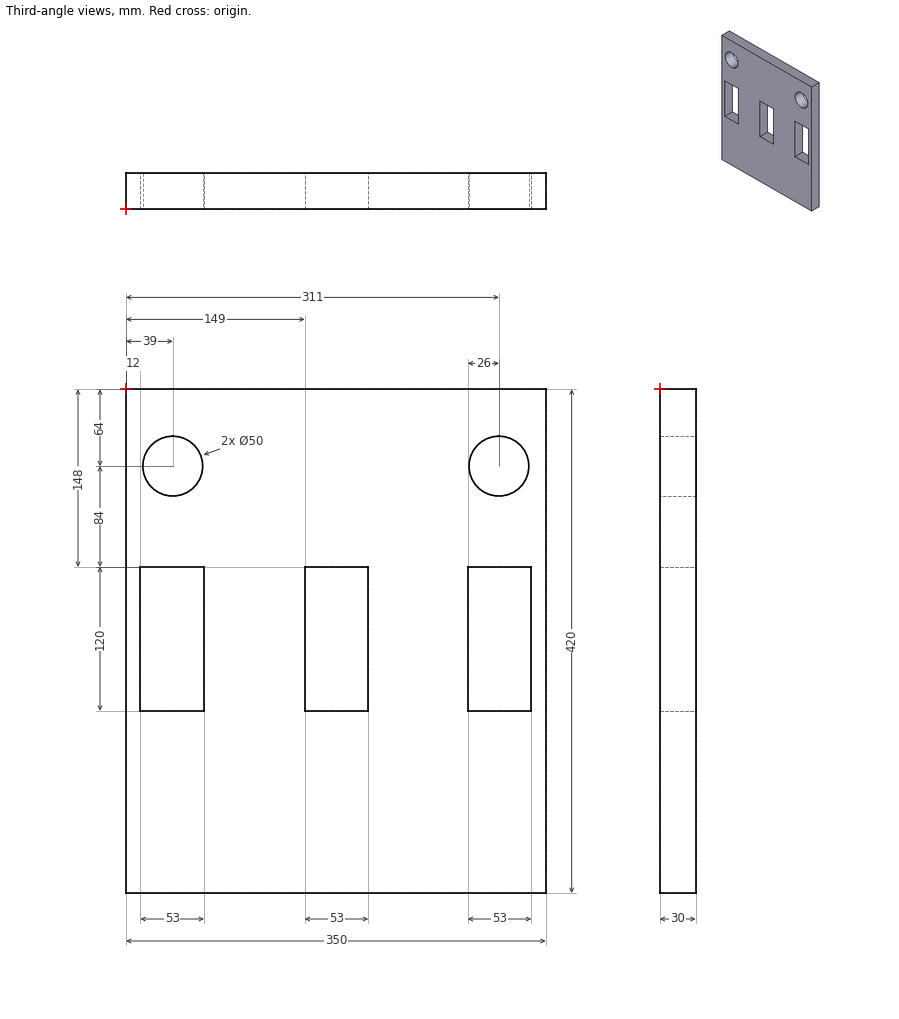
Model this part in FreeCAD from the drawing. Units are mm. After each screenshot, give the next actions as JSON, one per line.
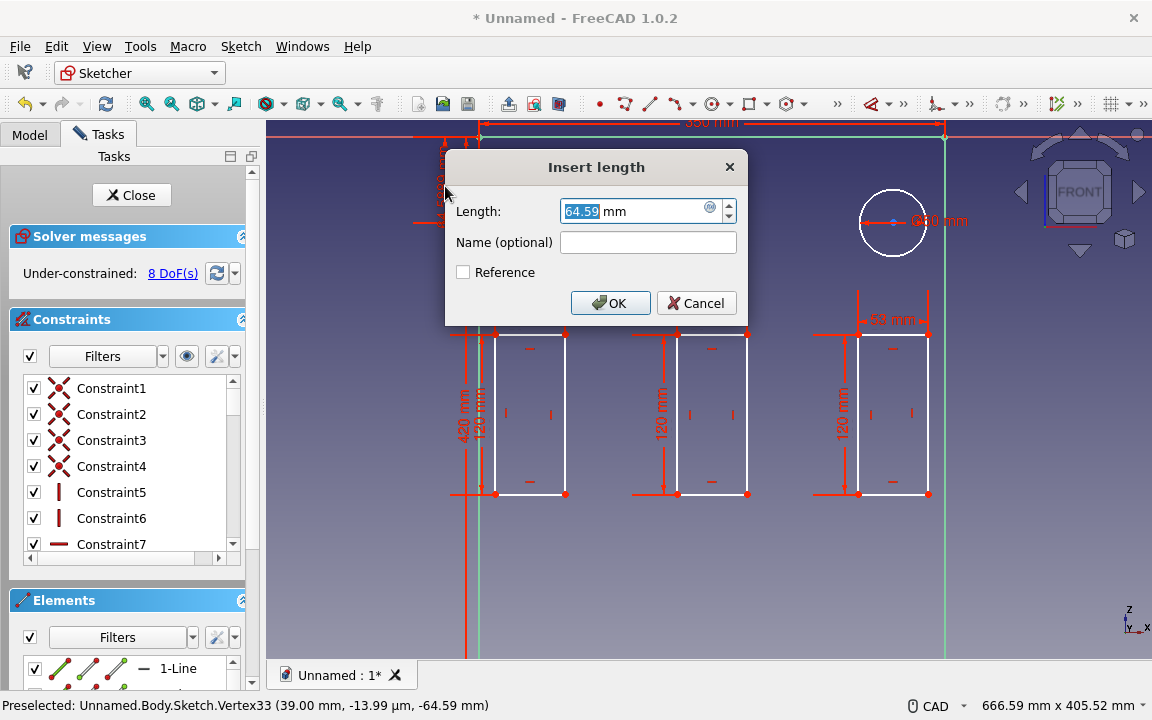
{"action": "type", "text": "64"}
{"action": "key", "text": "Return"}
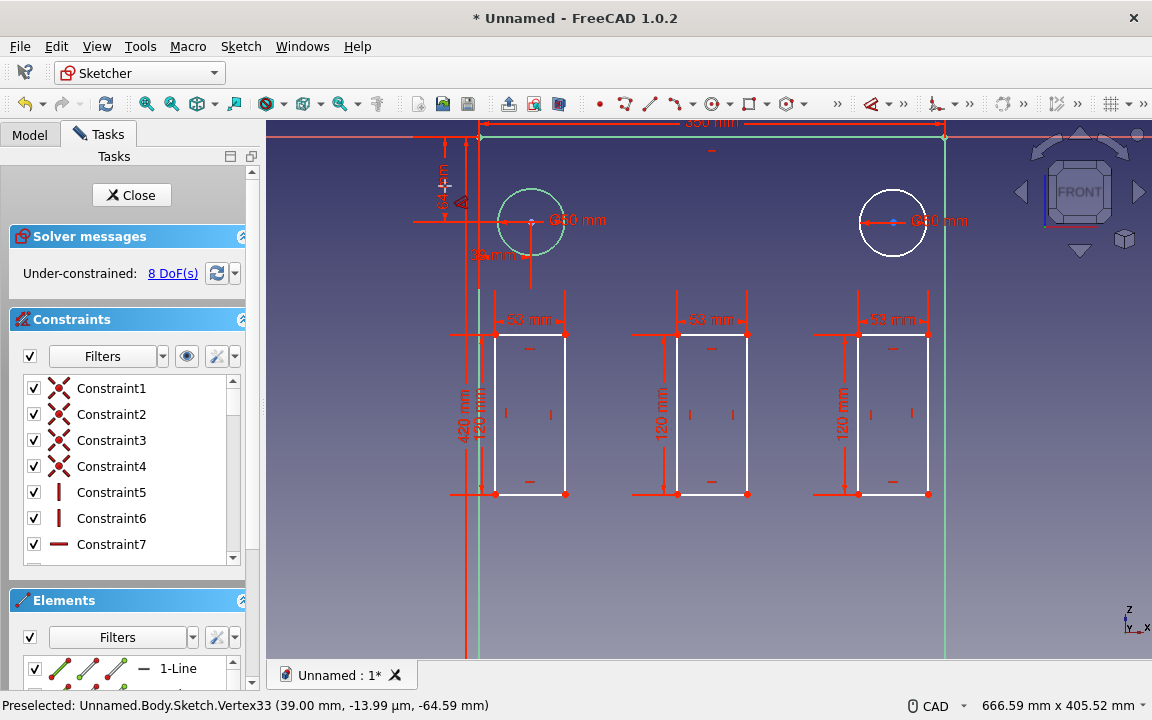
{"action": "left_click", "coordinate": [893, 223]}
{"action": "left_click", "coordinate": [445, 159]}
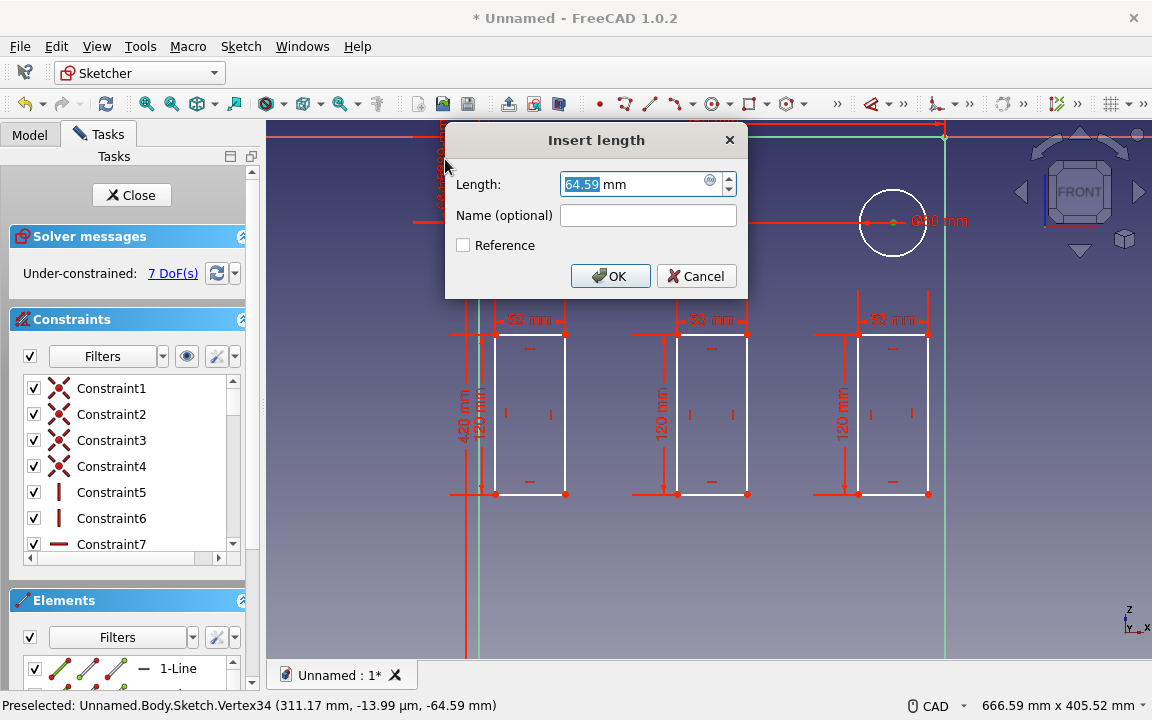
{"action": "type", "text": "64"}
{"action": "key", "text": "Return"}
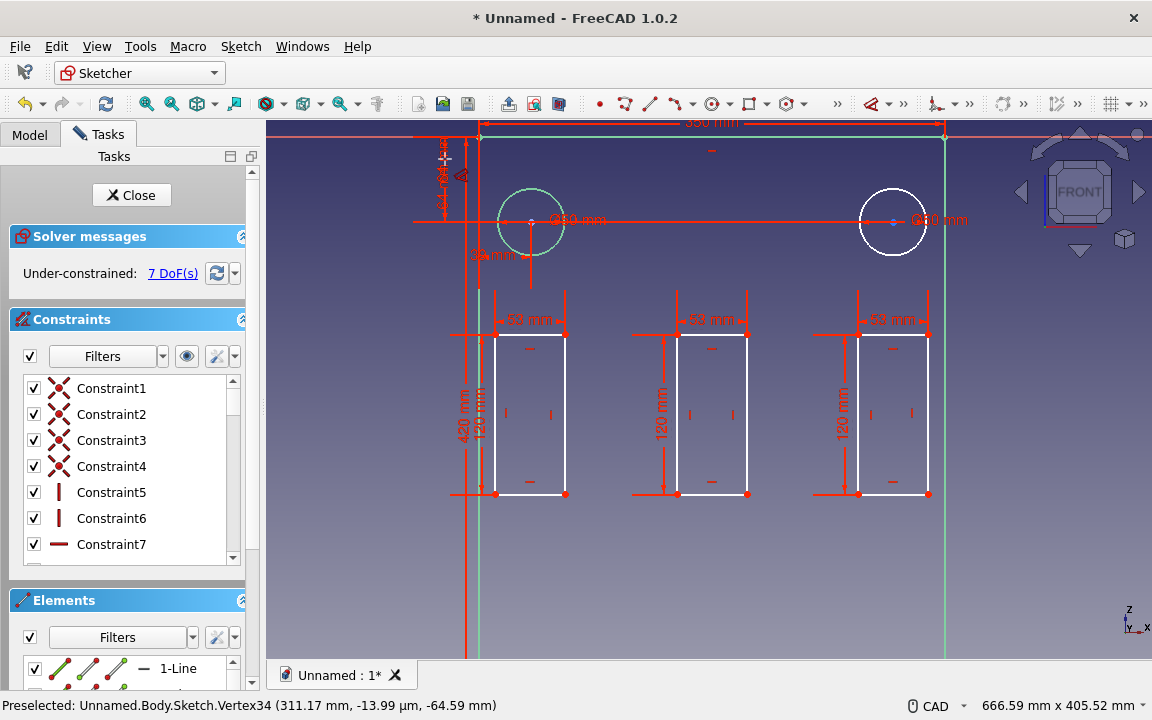
{"action": "scroll", "coordinate": [495, 335], "scroll_direction": "up", "scroll_amount": 5}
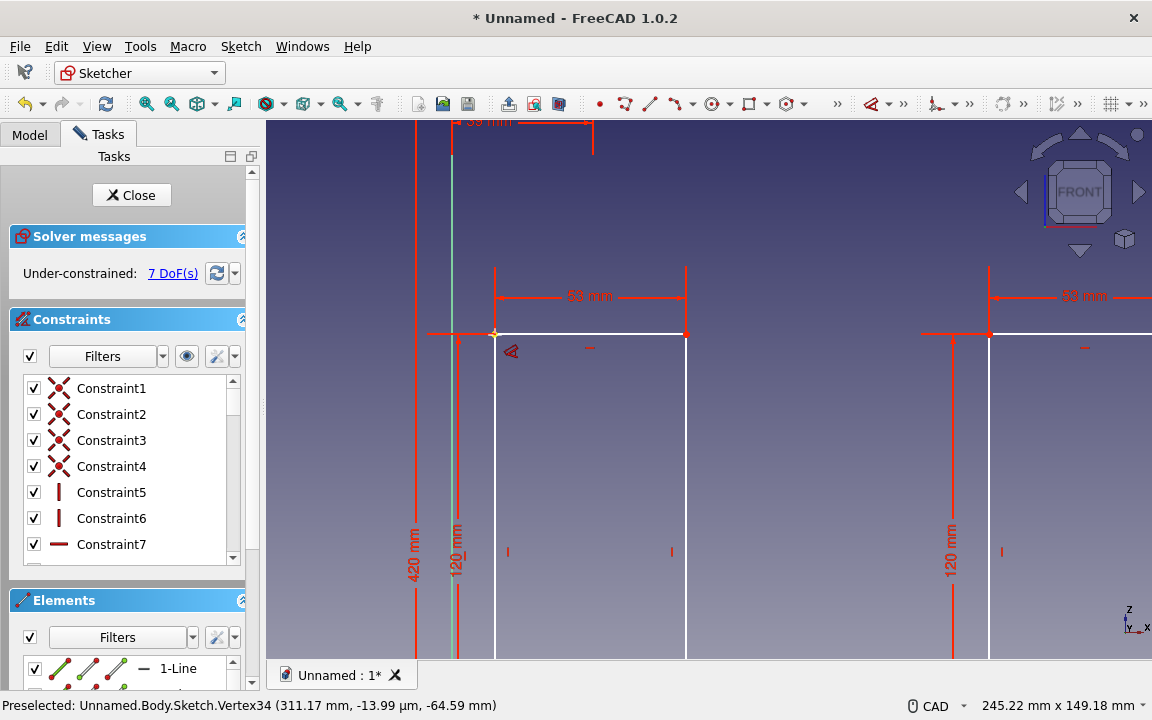
{"action": "left_click", "coordinate": [495, 334]}
{"action": "left_click", "coordinate": [473, 368]}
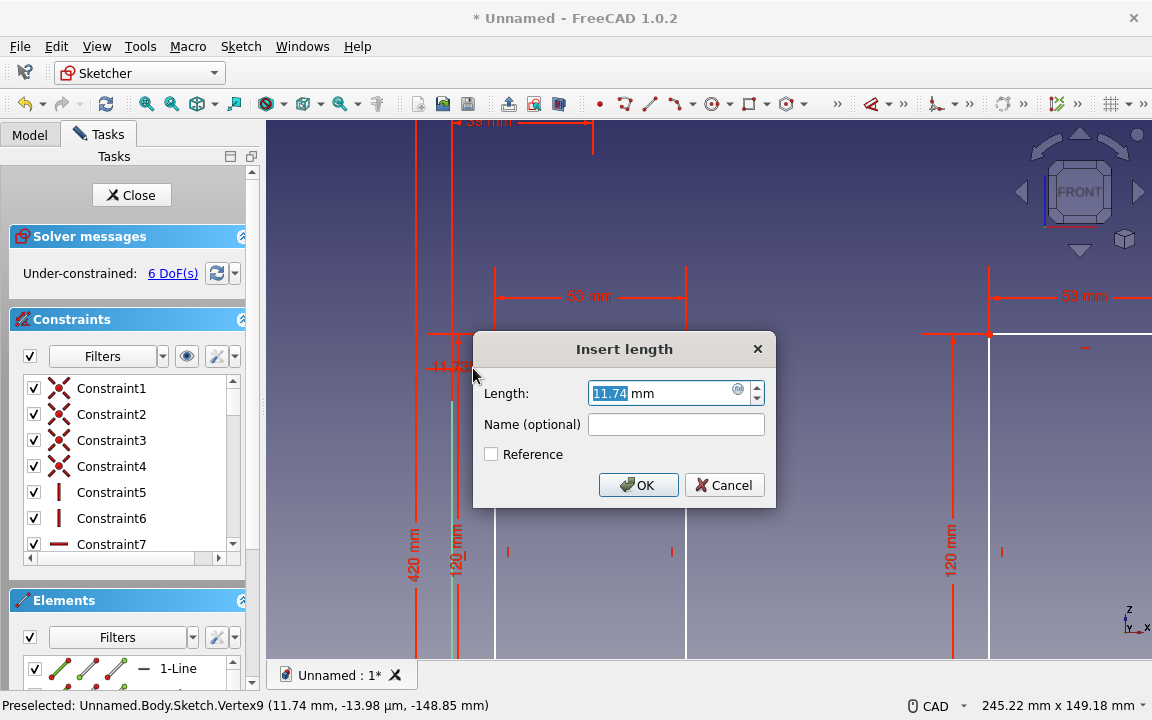
{"action": "type", "text": "12"}
{"action": "key", "text": "Return"}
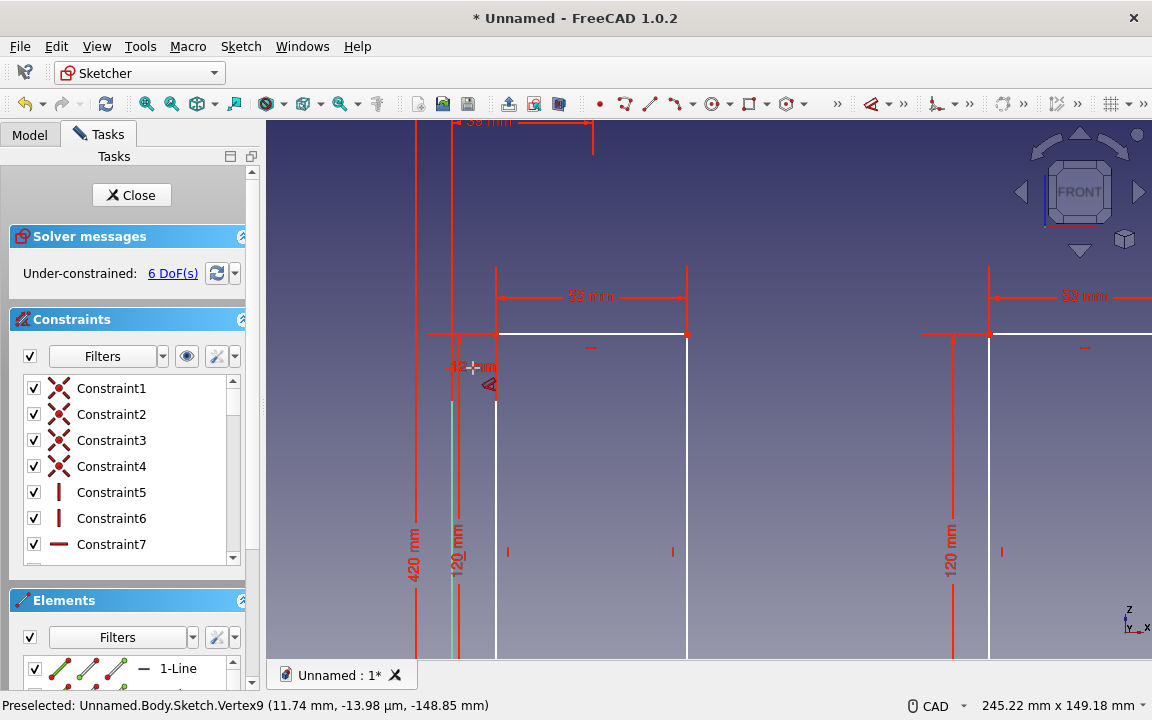
{"action": "scroll", "coordinate": [495, 335], "scroll_direction": "down", "scroll_amount": 7}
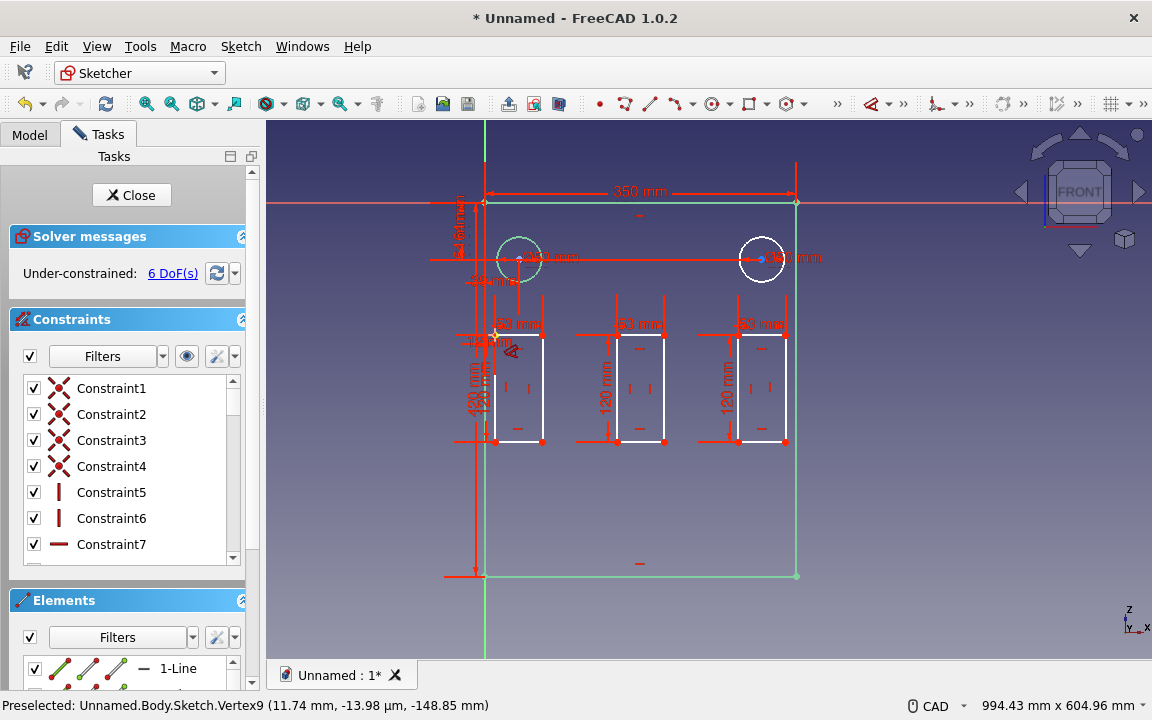
{"action": "left_click", "coordinate": [762, 260]}
{"action": "left_click", "coordinate": [623, 169]}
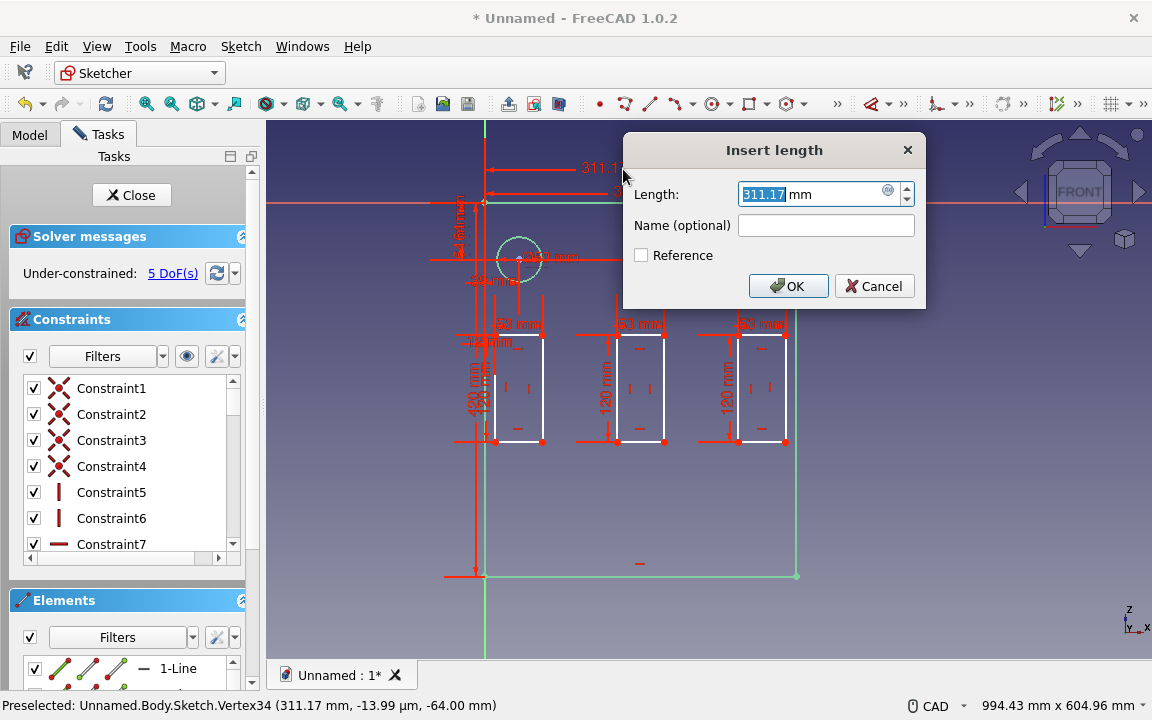
{"action": "type", "text": "311"}
{"action": "key", "text": "Return"}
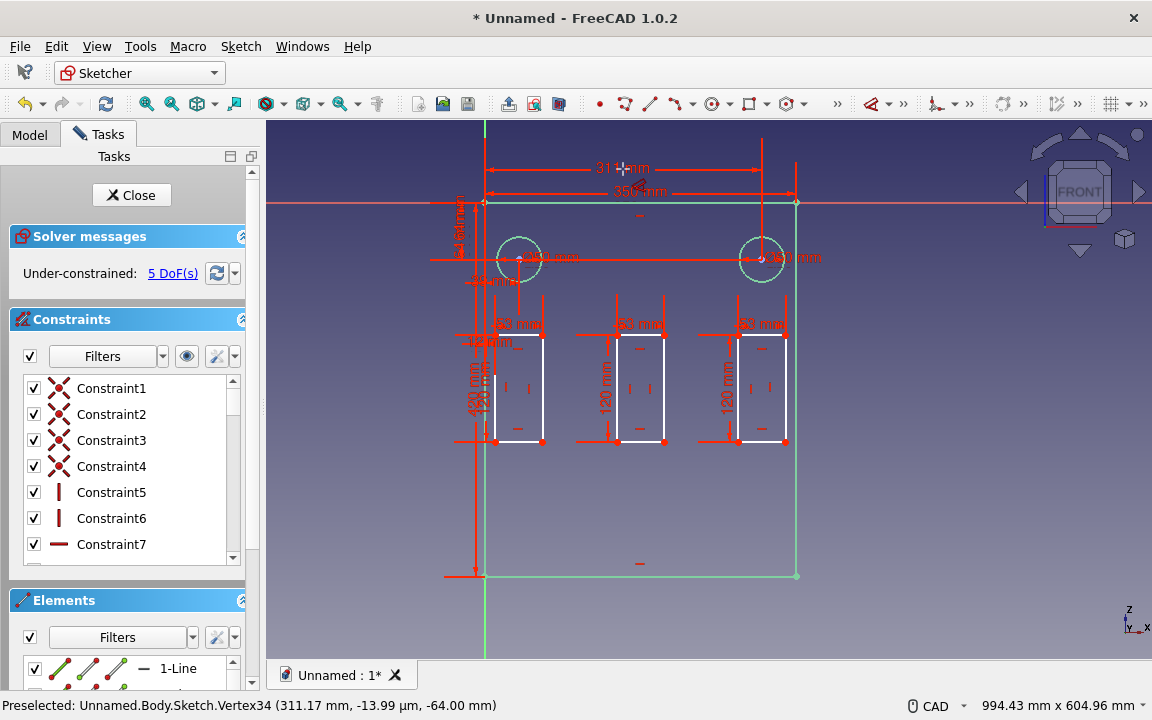
{"action": "left_click", "coordinate": [543, 335]}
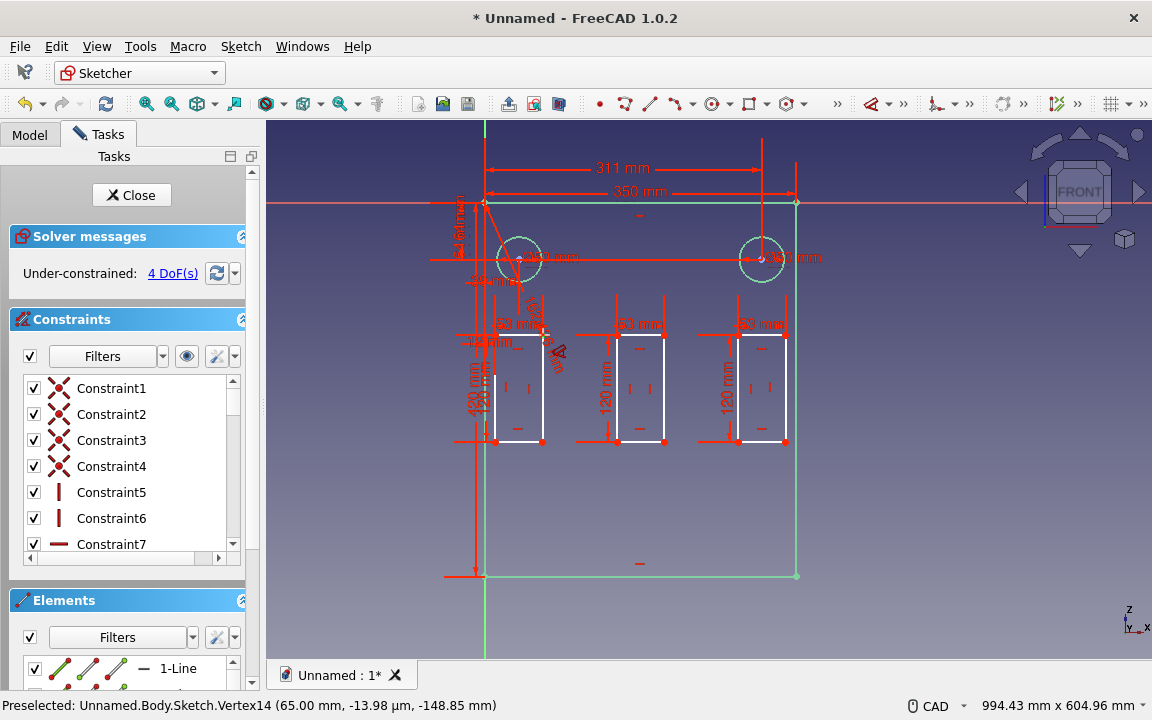
{"action": "left_click", "coordinate": [519, 260]}
{"action": "left_click", "coordinate": [577, 297]}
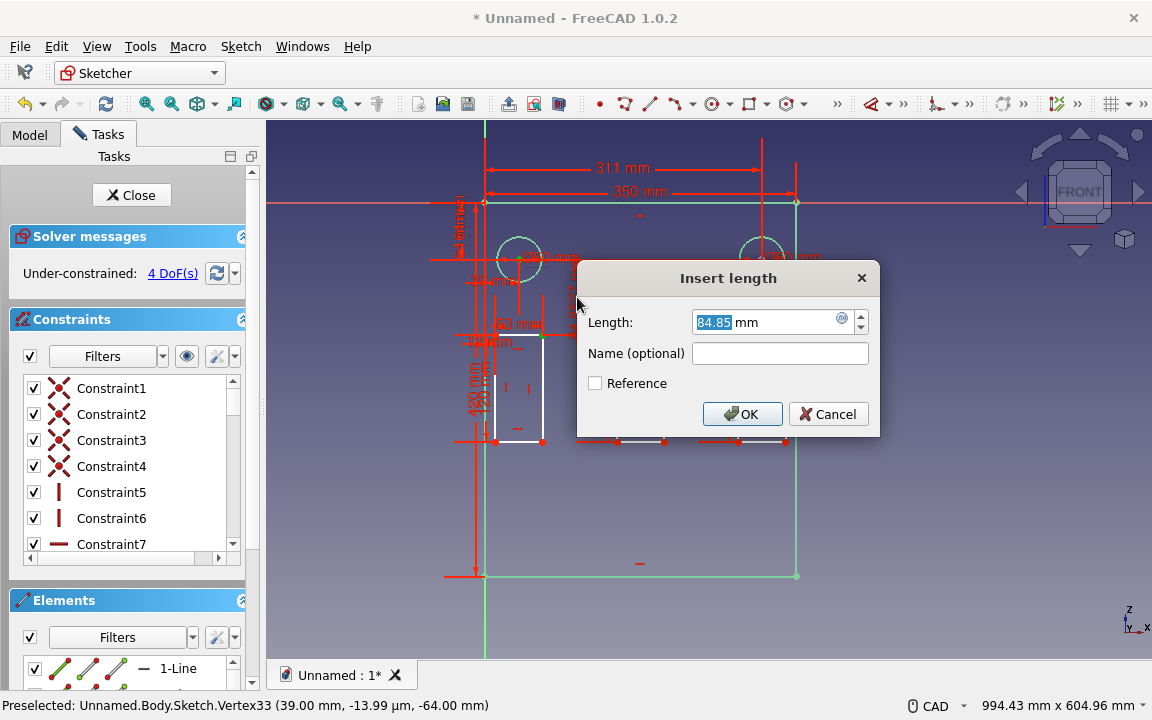
{"action": "type", "text": "84"}
{"action": "key", "text": "Return"}